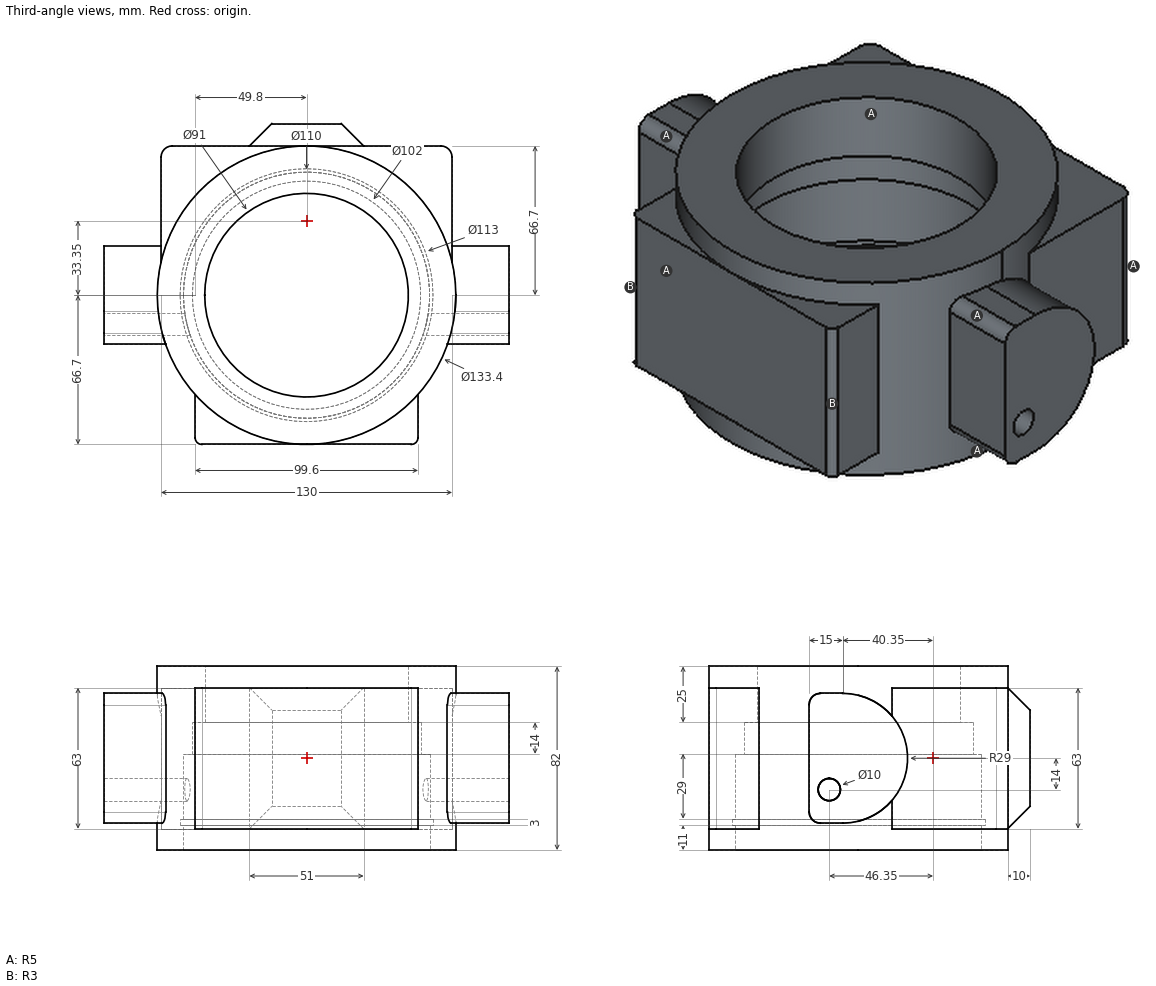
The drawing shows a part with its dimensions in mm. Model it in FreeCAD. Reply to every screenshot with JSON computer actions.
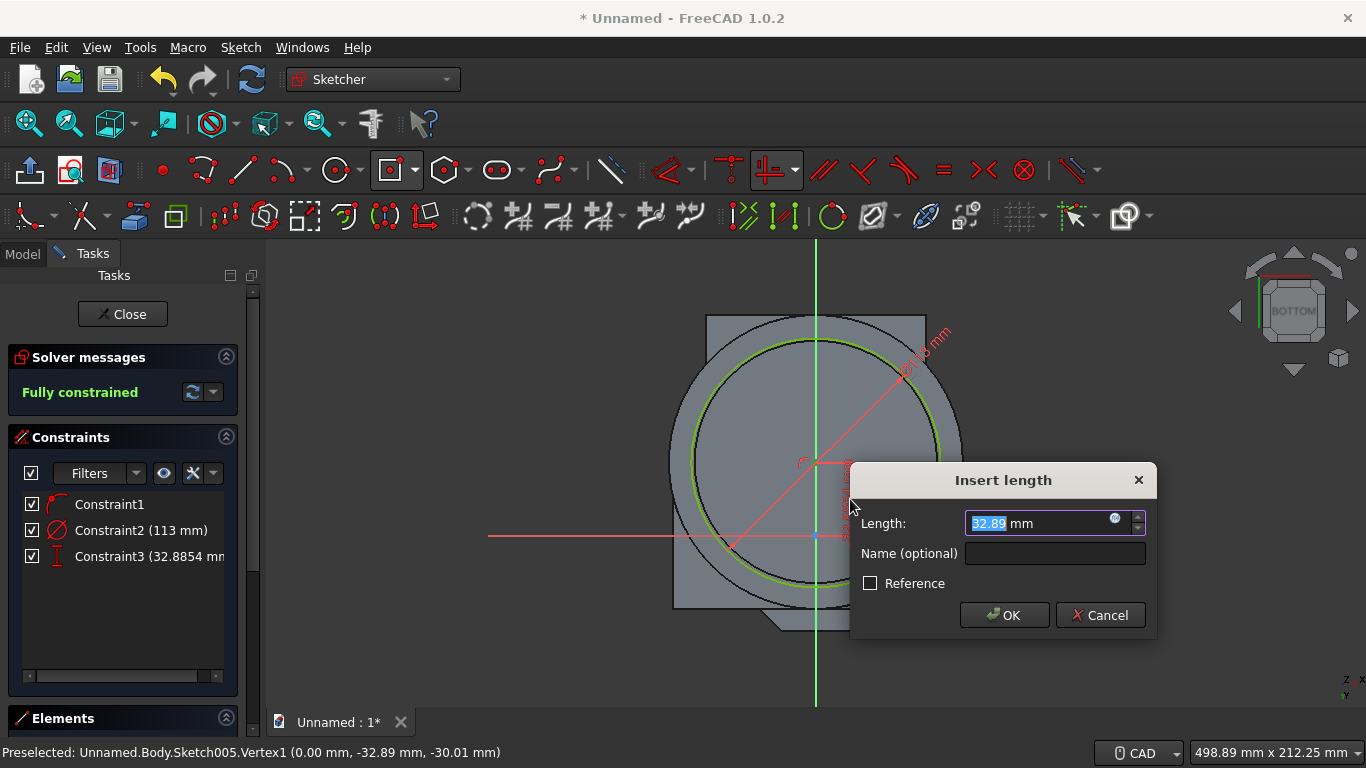
{"action": "type", "text": "33.35"}
{"action": "key", "text": "Return"}
{"action": "key", "text": "Escape"}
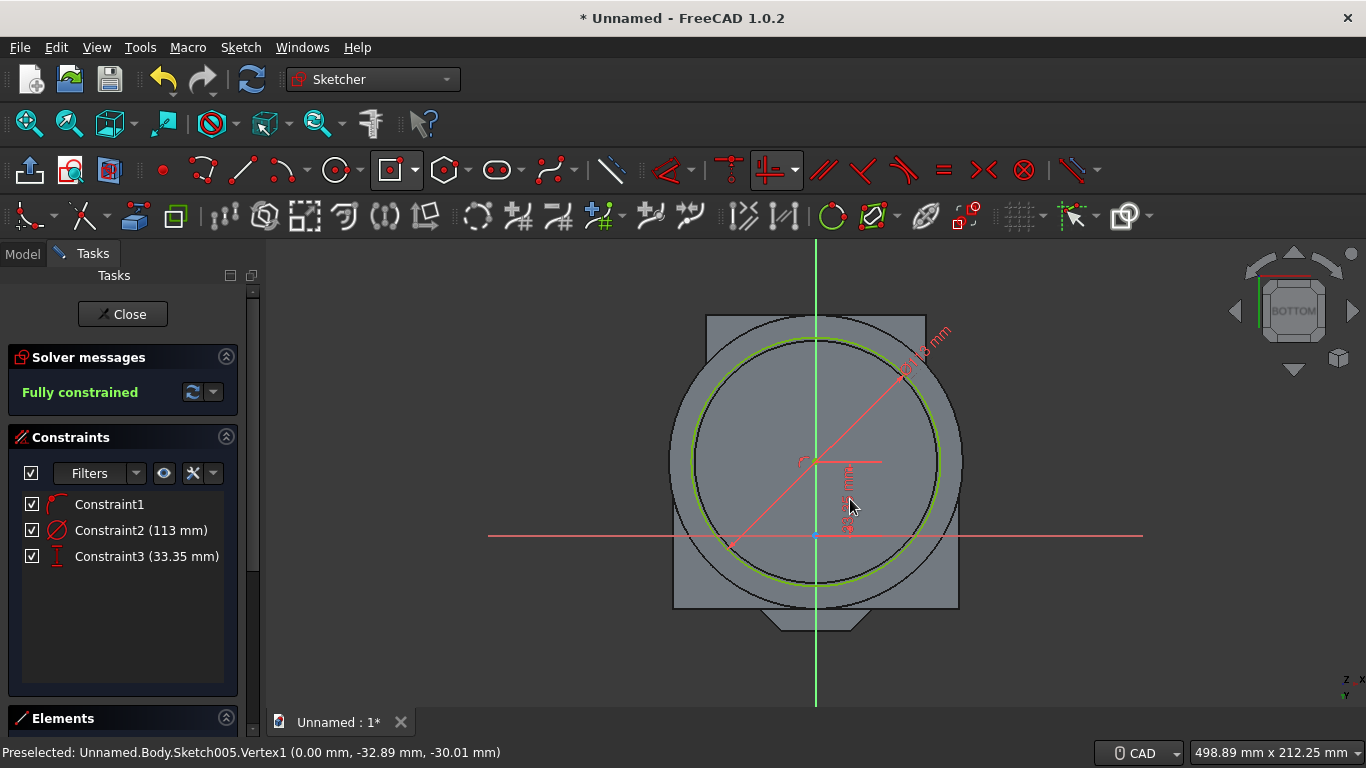
{"action": "left_click", "coordinate": [123, 314]}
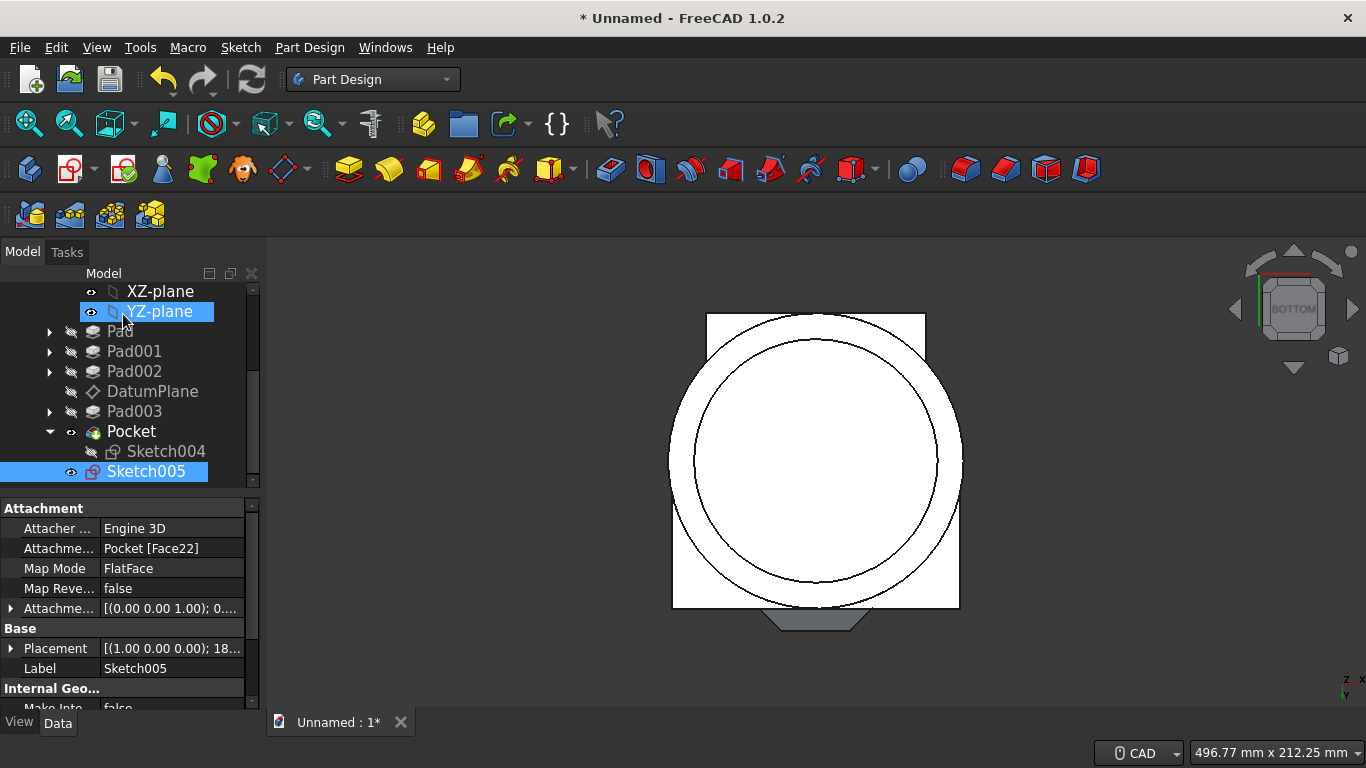
{"action": "left_click", "coordinate": [612, 170]}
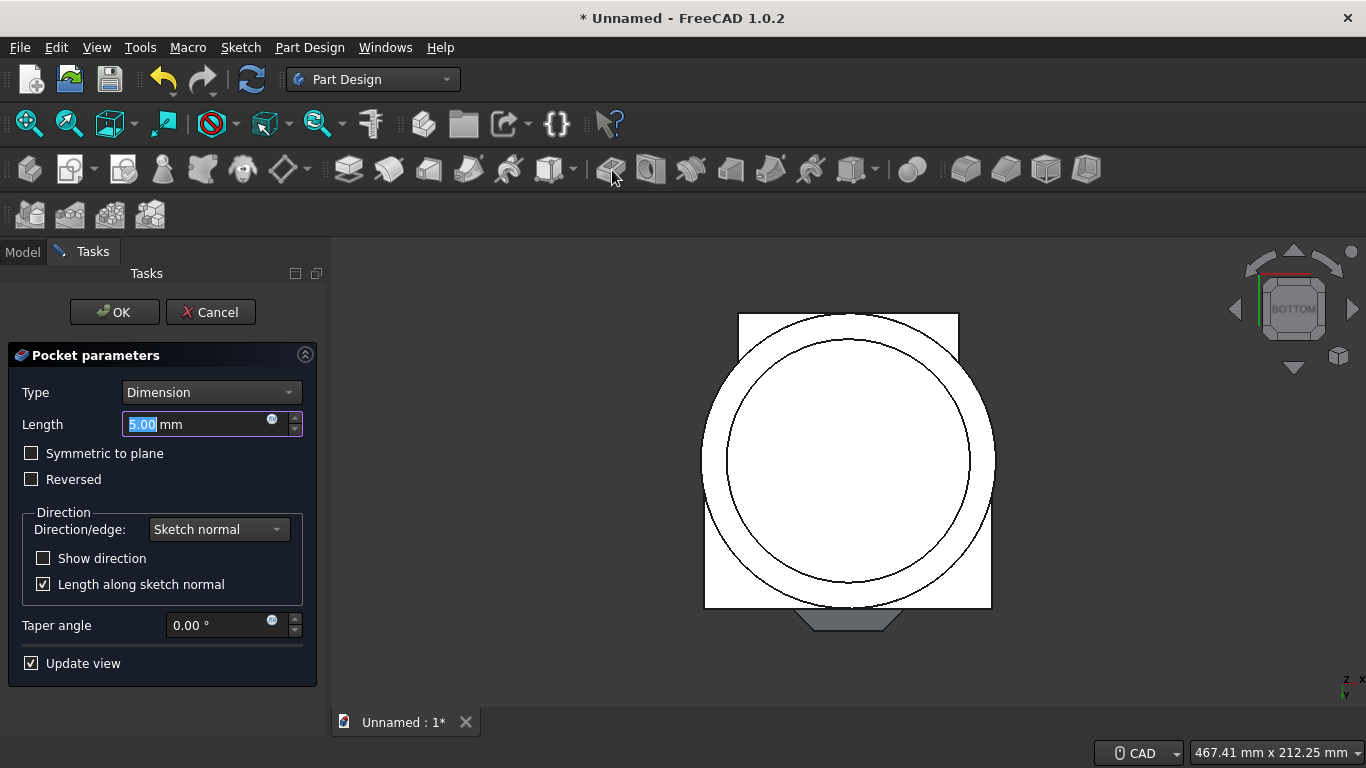
{"action": "type", "text": "3"}
{"action": "key", "text": "Tab"}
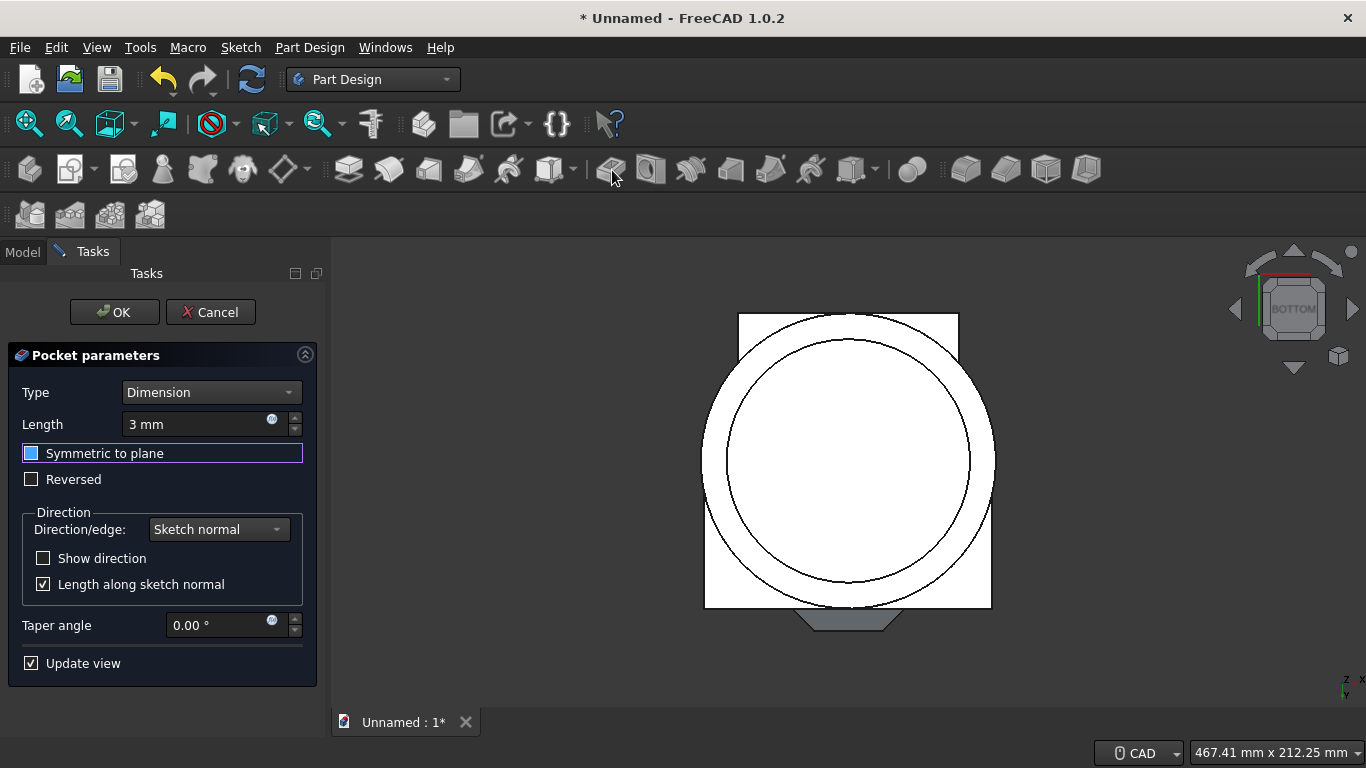
{"action": "left_click", "coordinate": [115, 312]}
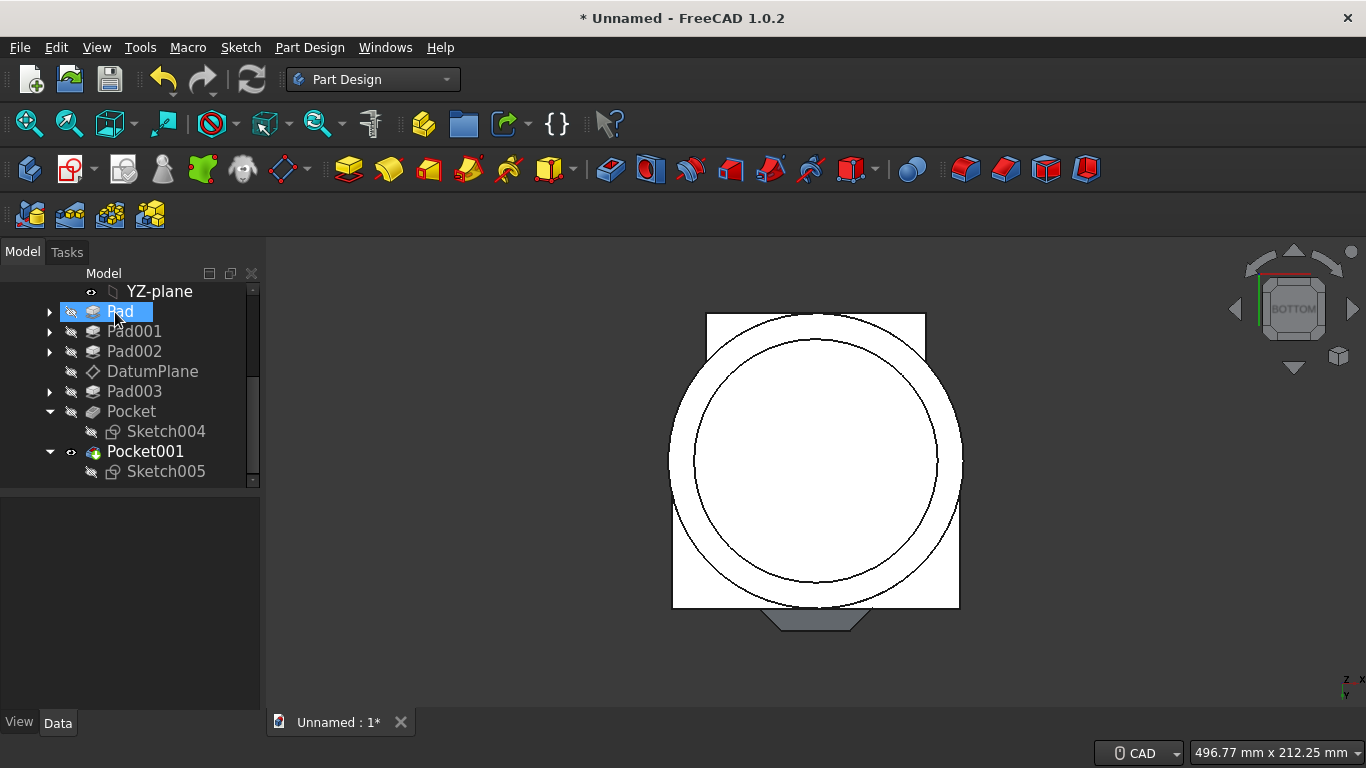
{"action": "left_click", "coordinate": [816, 460]}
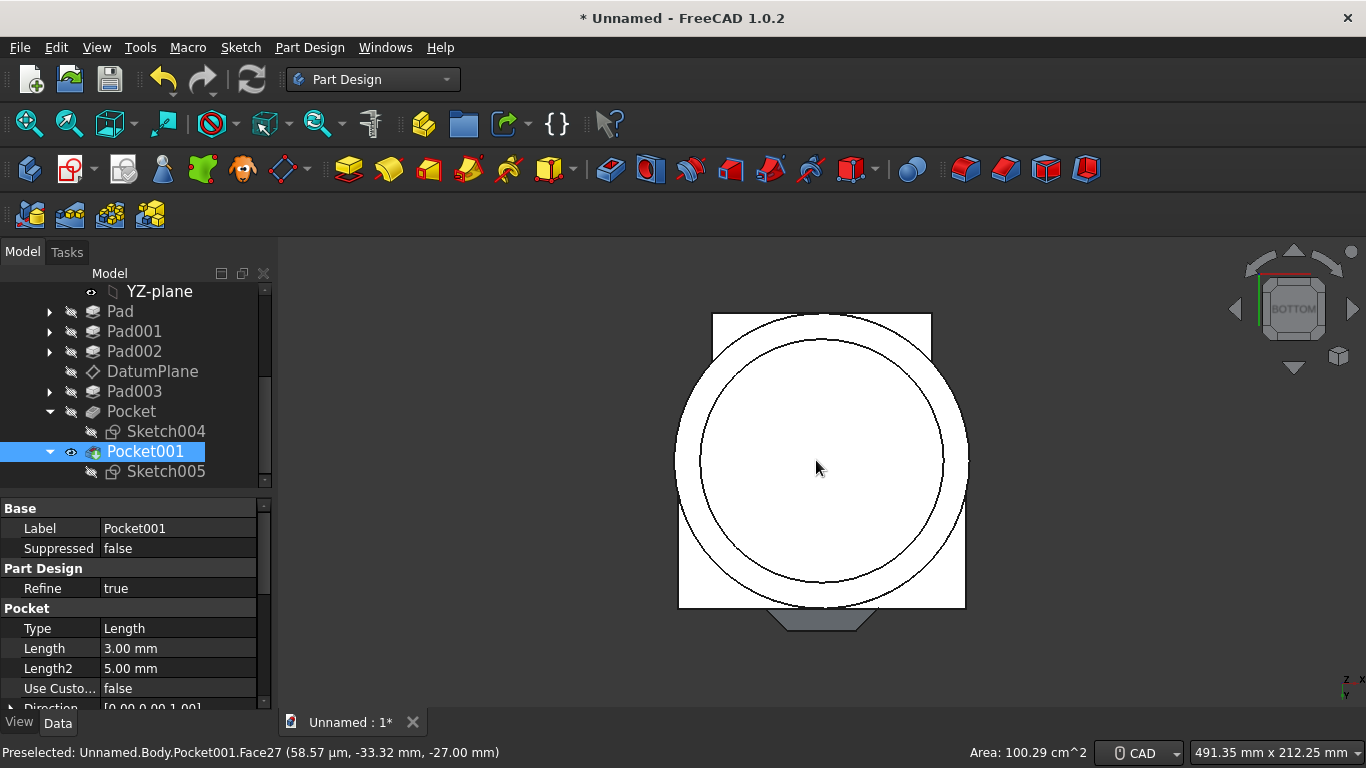
{"action": "left_click", "coordinate": [70, 170]}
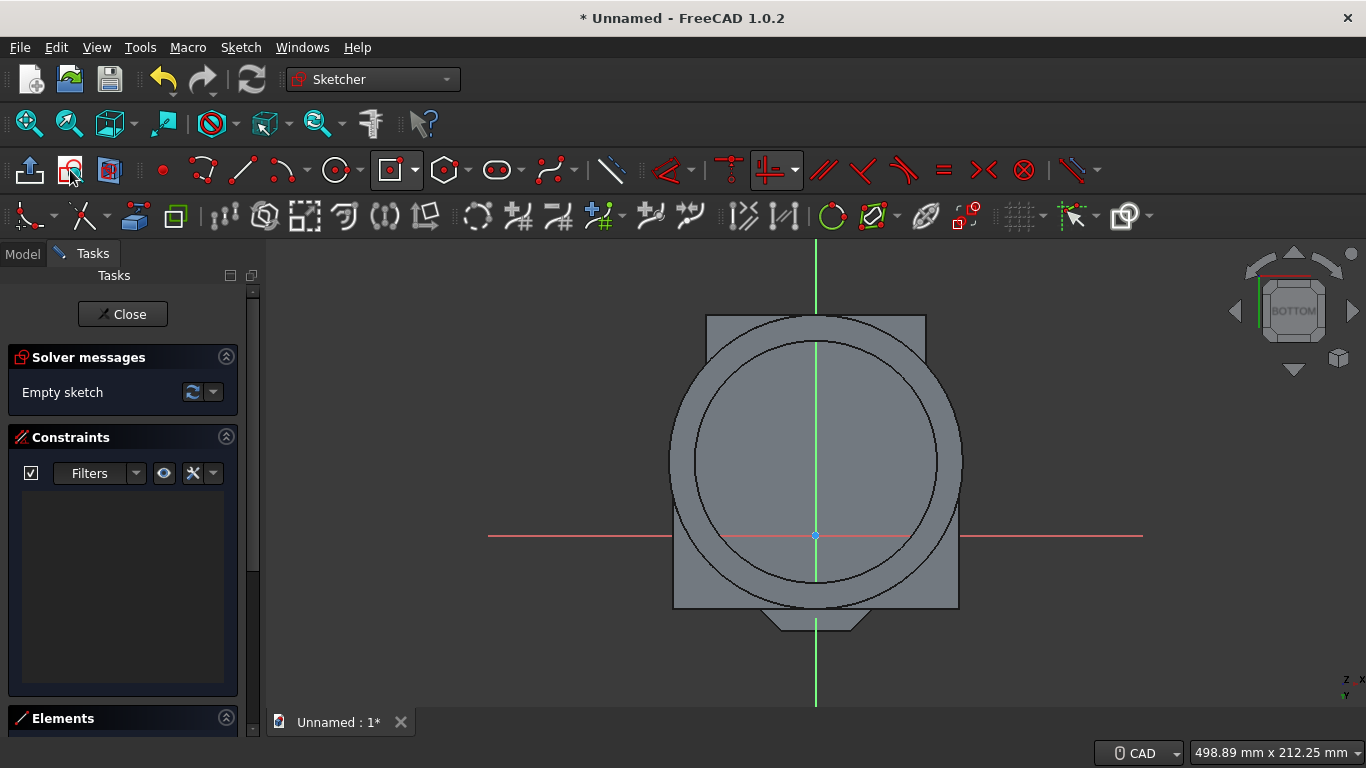
{"action": "key", "text": "q s"}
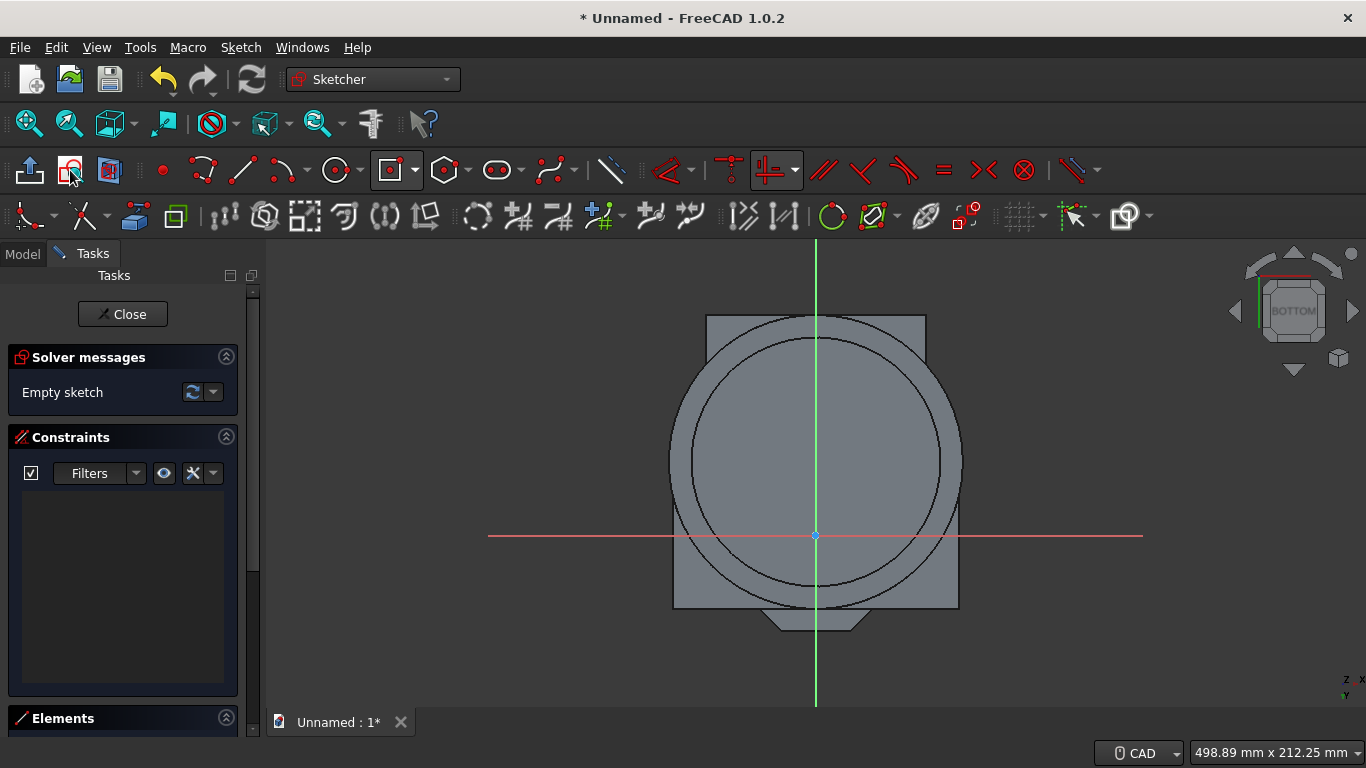
{"action": "key", "text": "g c"}